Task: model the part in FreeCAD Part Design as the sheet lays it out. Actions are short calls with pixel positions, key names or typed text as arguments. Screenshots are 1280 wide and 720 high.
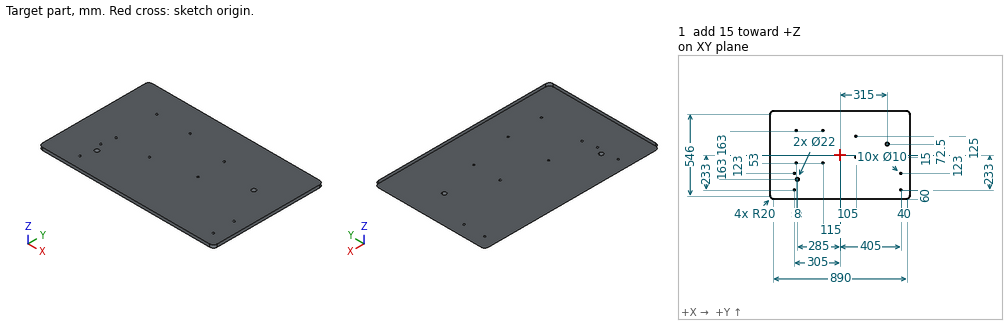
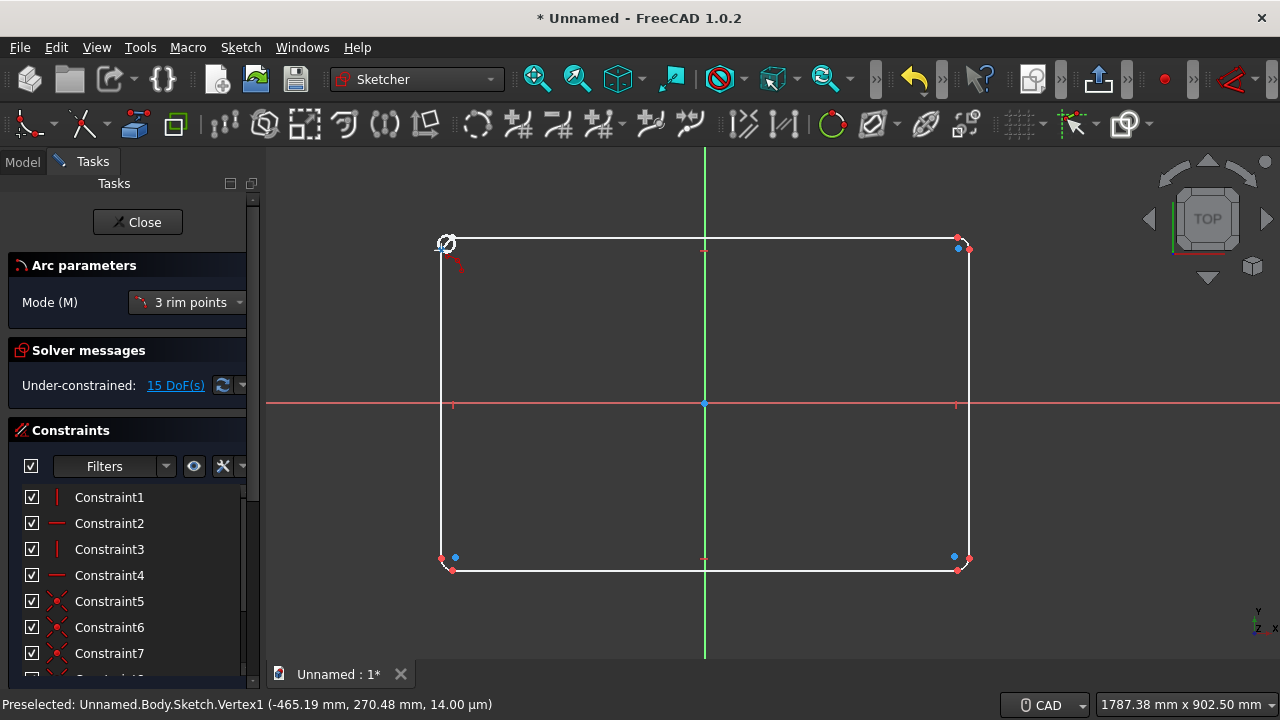
scroll(444, 241, up, 8)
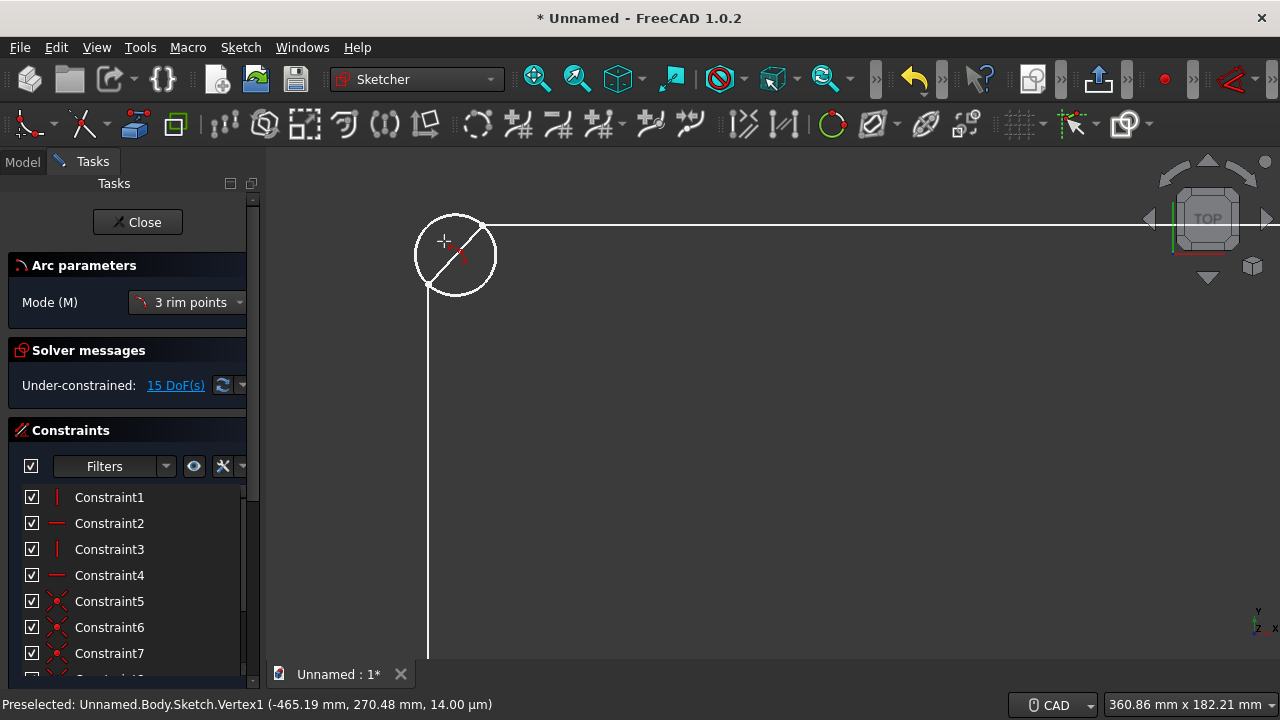
click(445, 238)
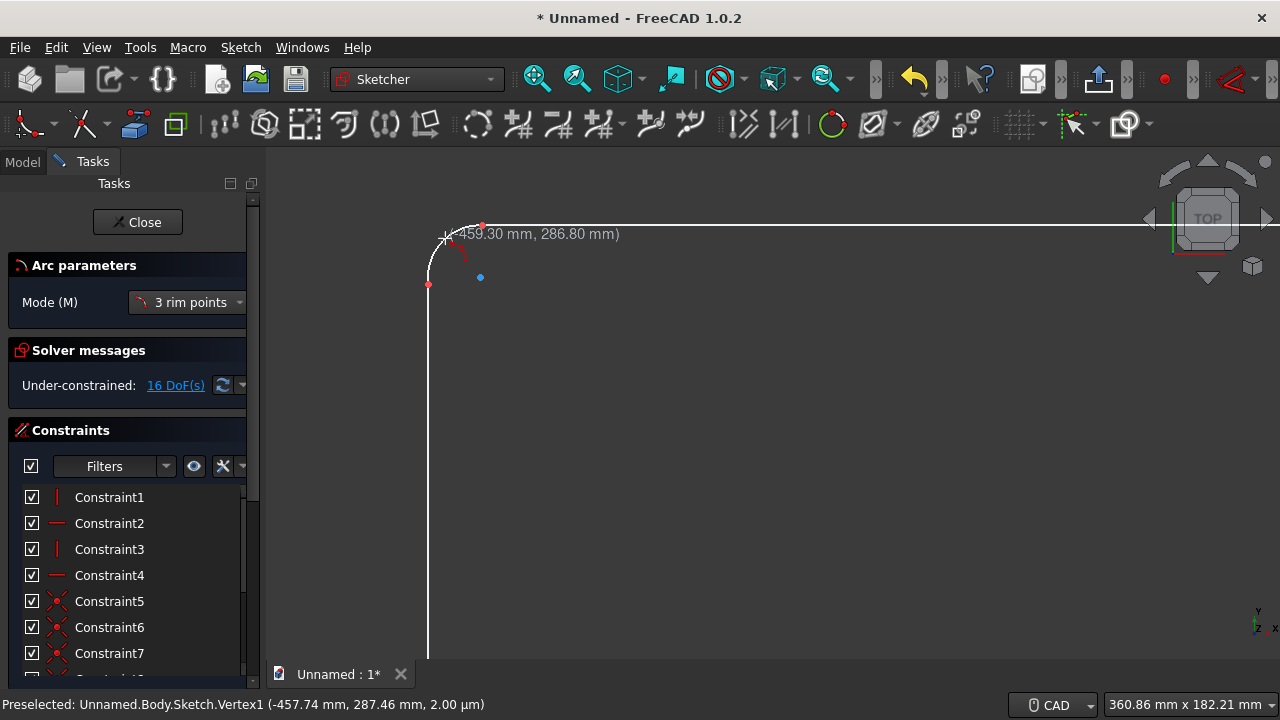
key(g)
key(c)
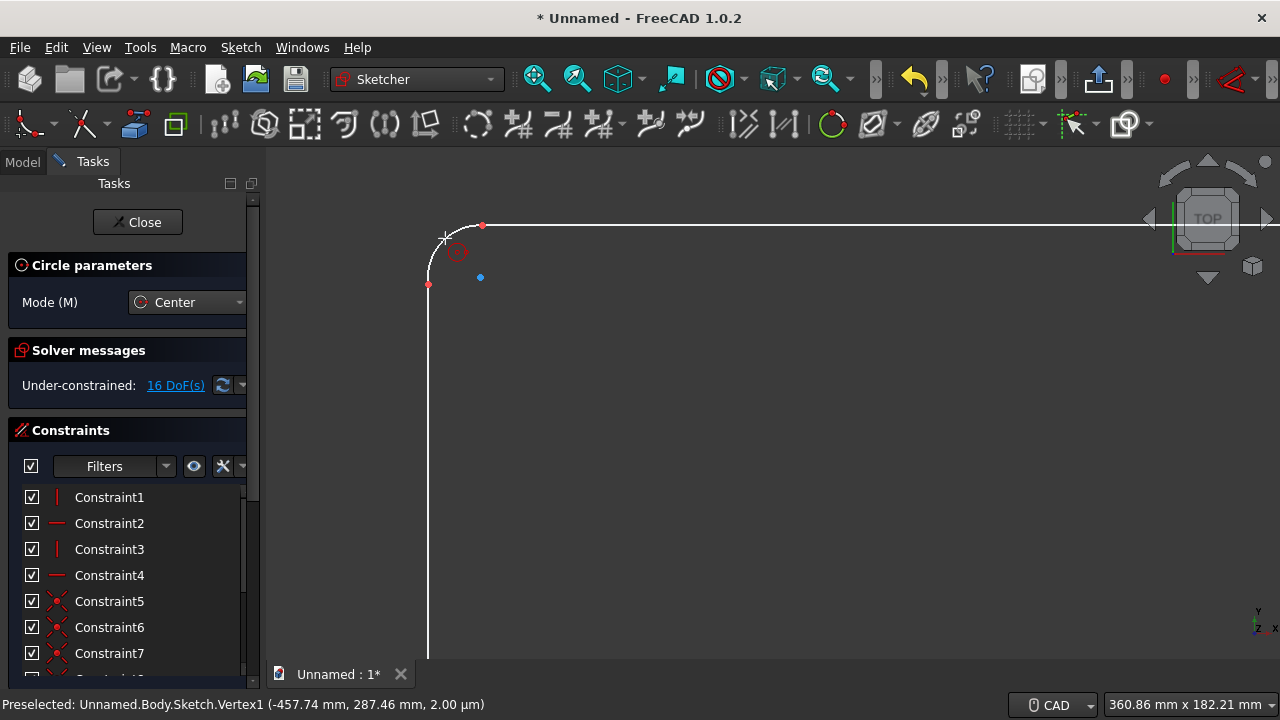
scroll(444, 241, down, 8)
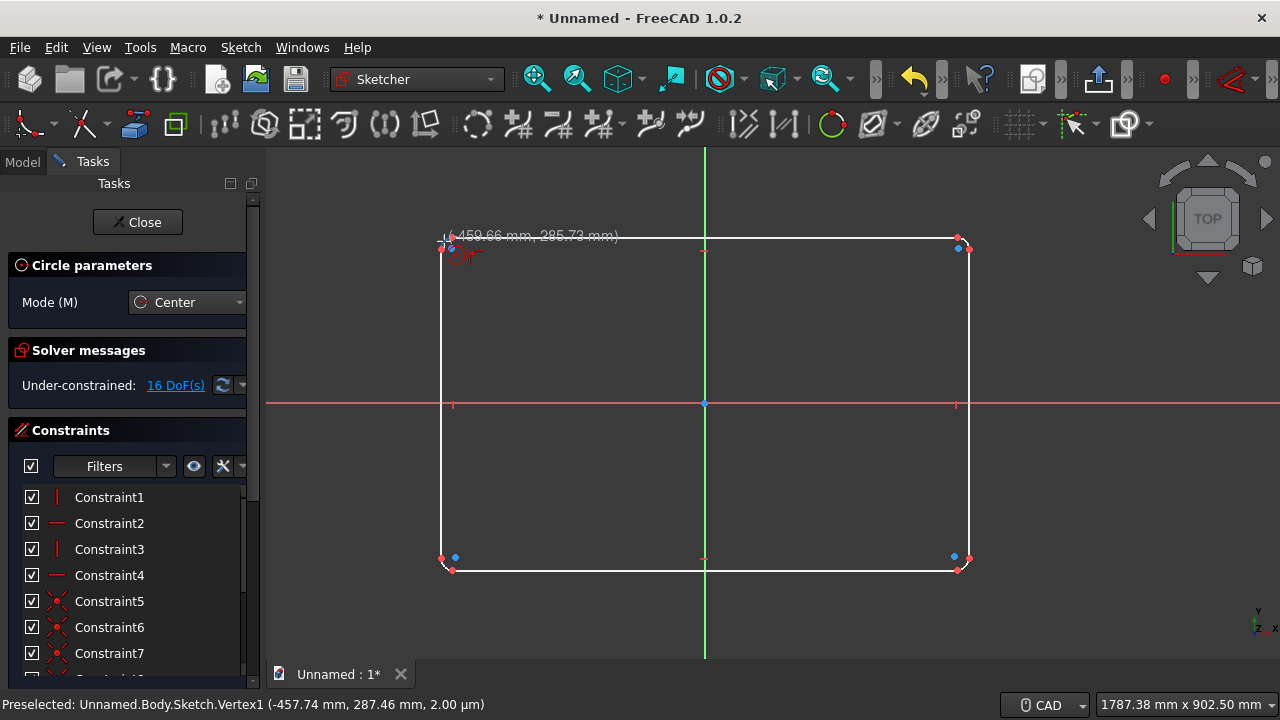
scroll(935, 536, up, 11)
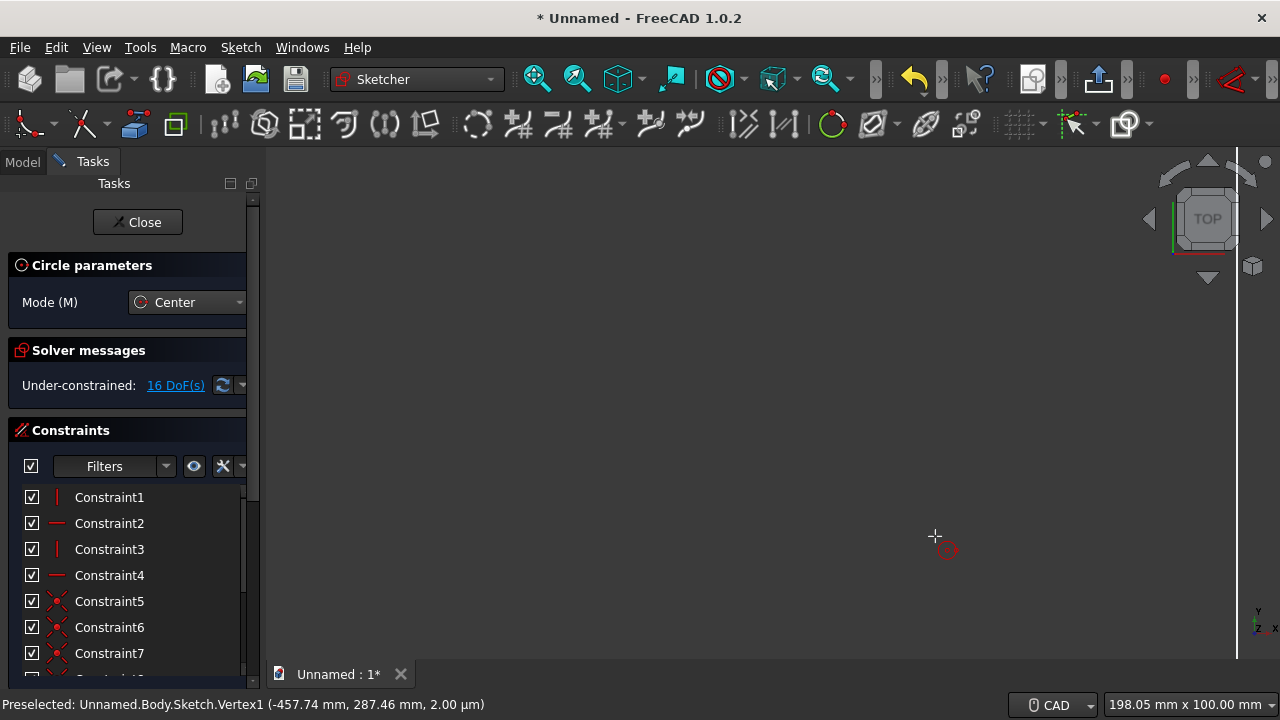
scroll(935, 536, down, 11)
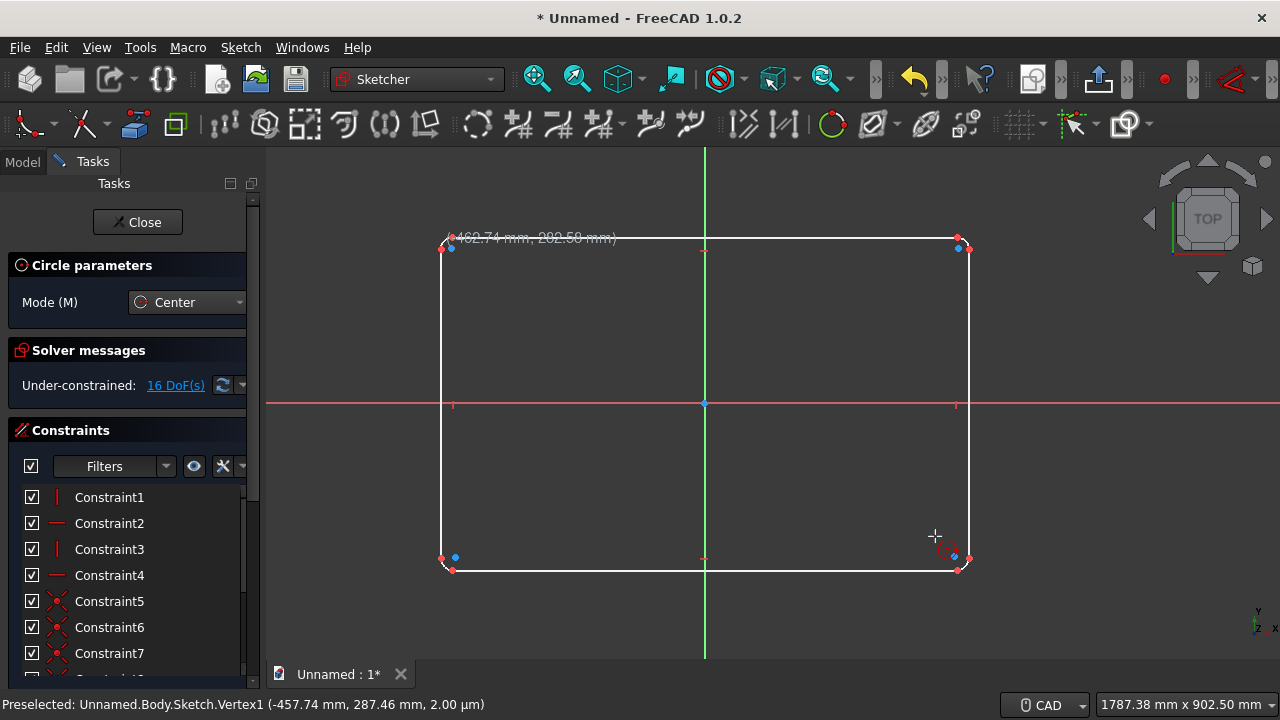
click(935, 536)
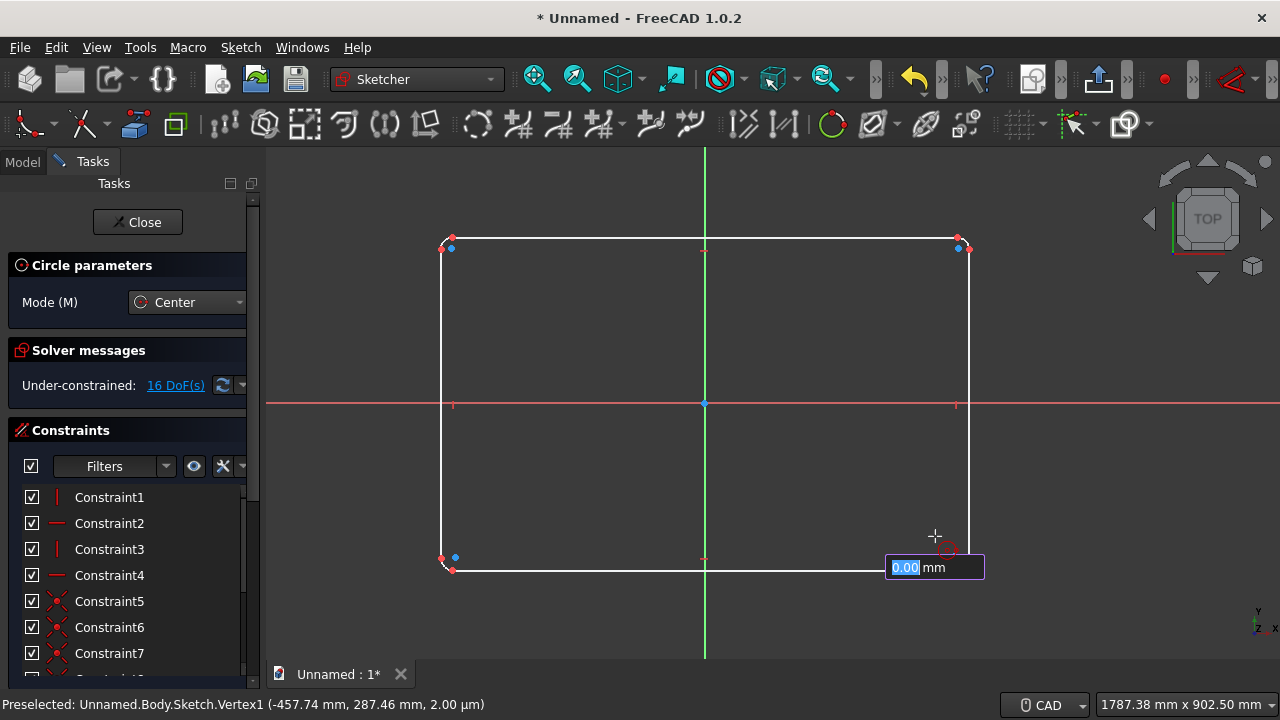
scroll(937, 534, up, 9)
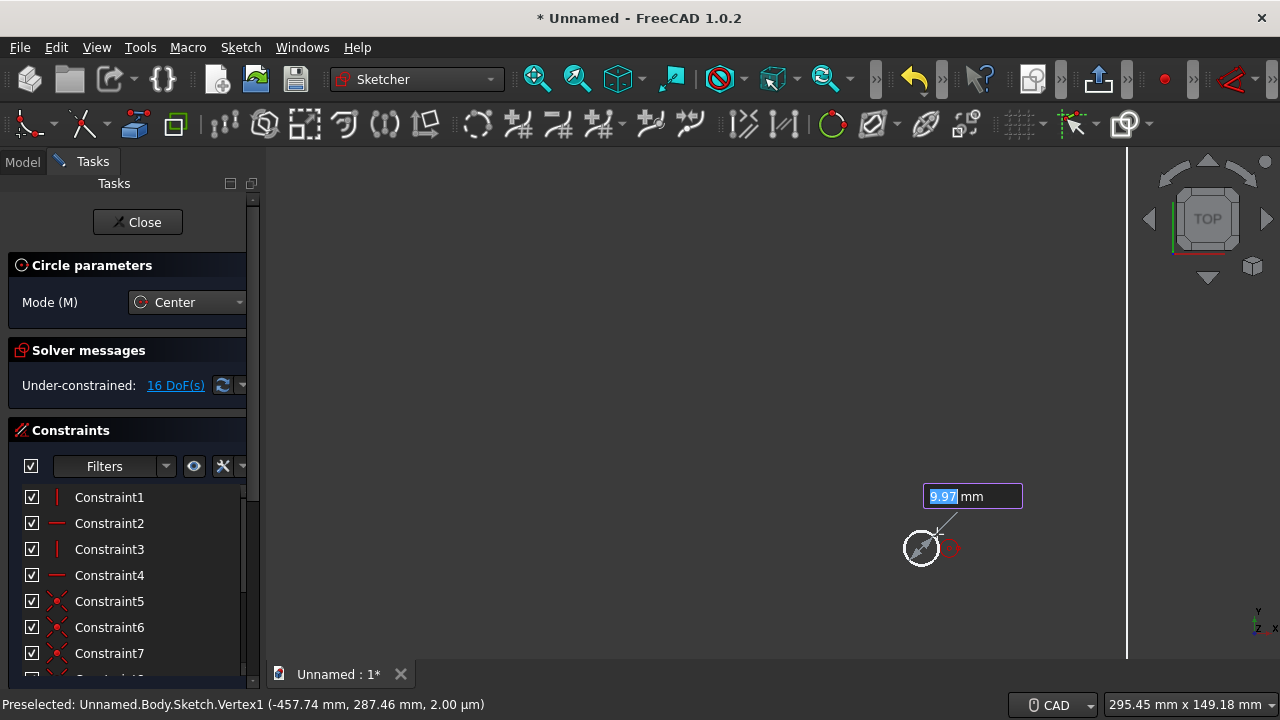
click(932, 528)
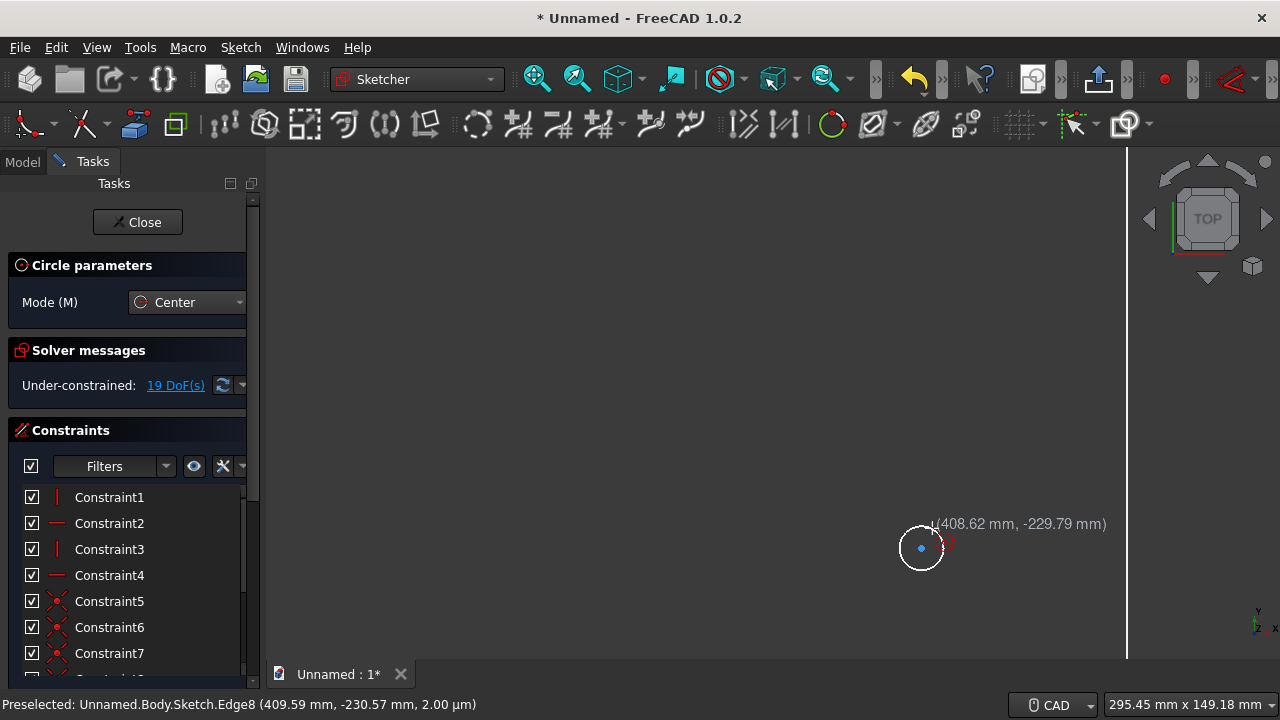
scroll(937, 534, down, 9)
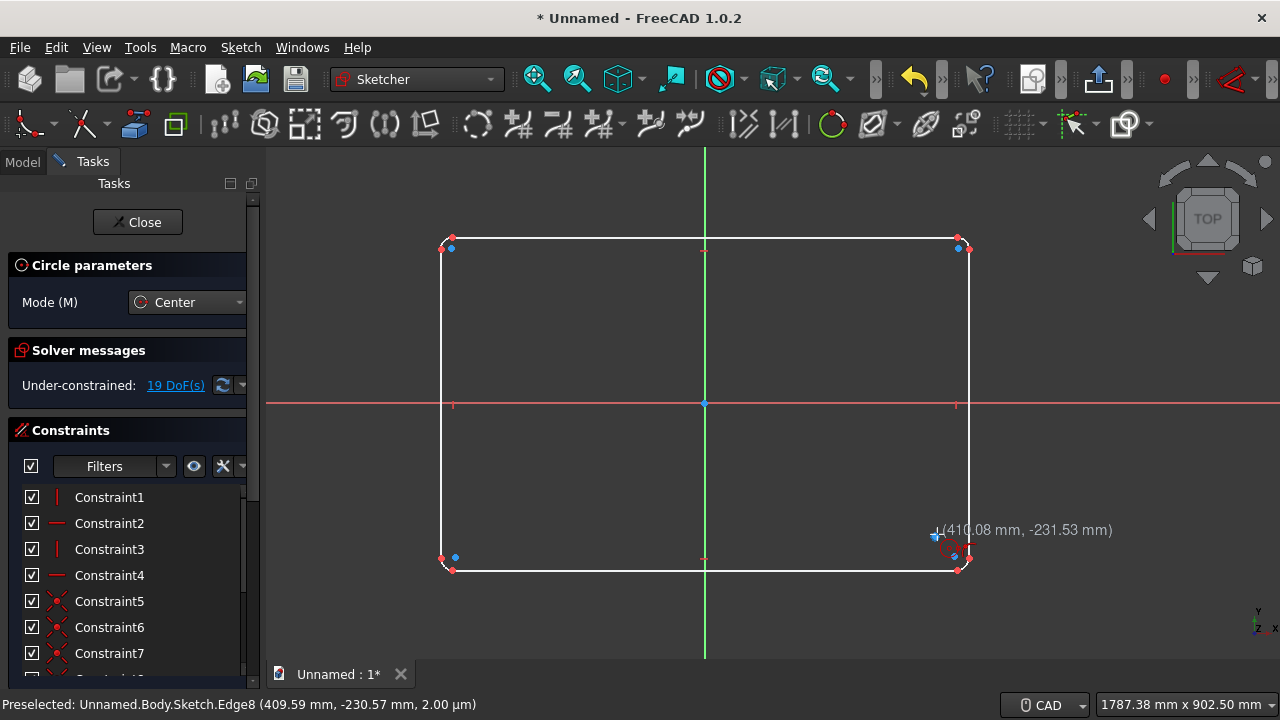
scroll(935, 473, up, 11)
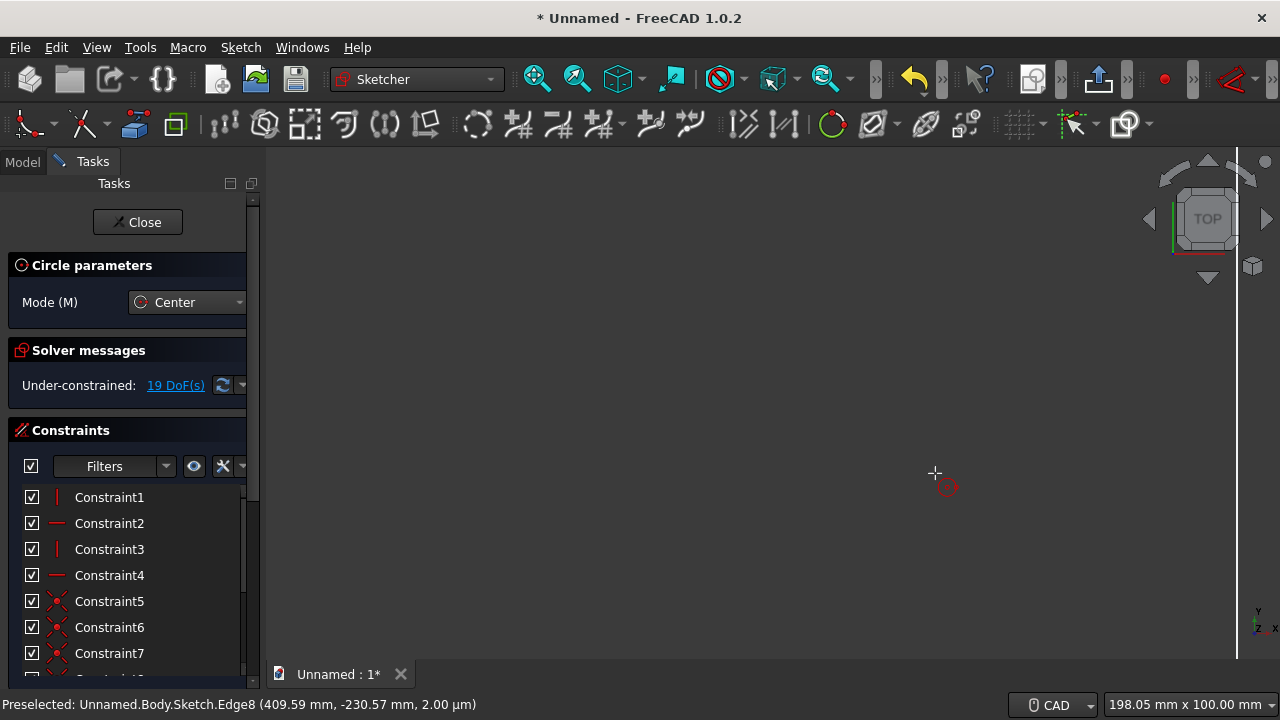
scroll(935, 473, down, 11)